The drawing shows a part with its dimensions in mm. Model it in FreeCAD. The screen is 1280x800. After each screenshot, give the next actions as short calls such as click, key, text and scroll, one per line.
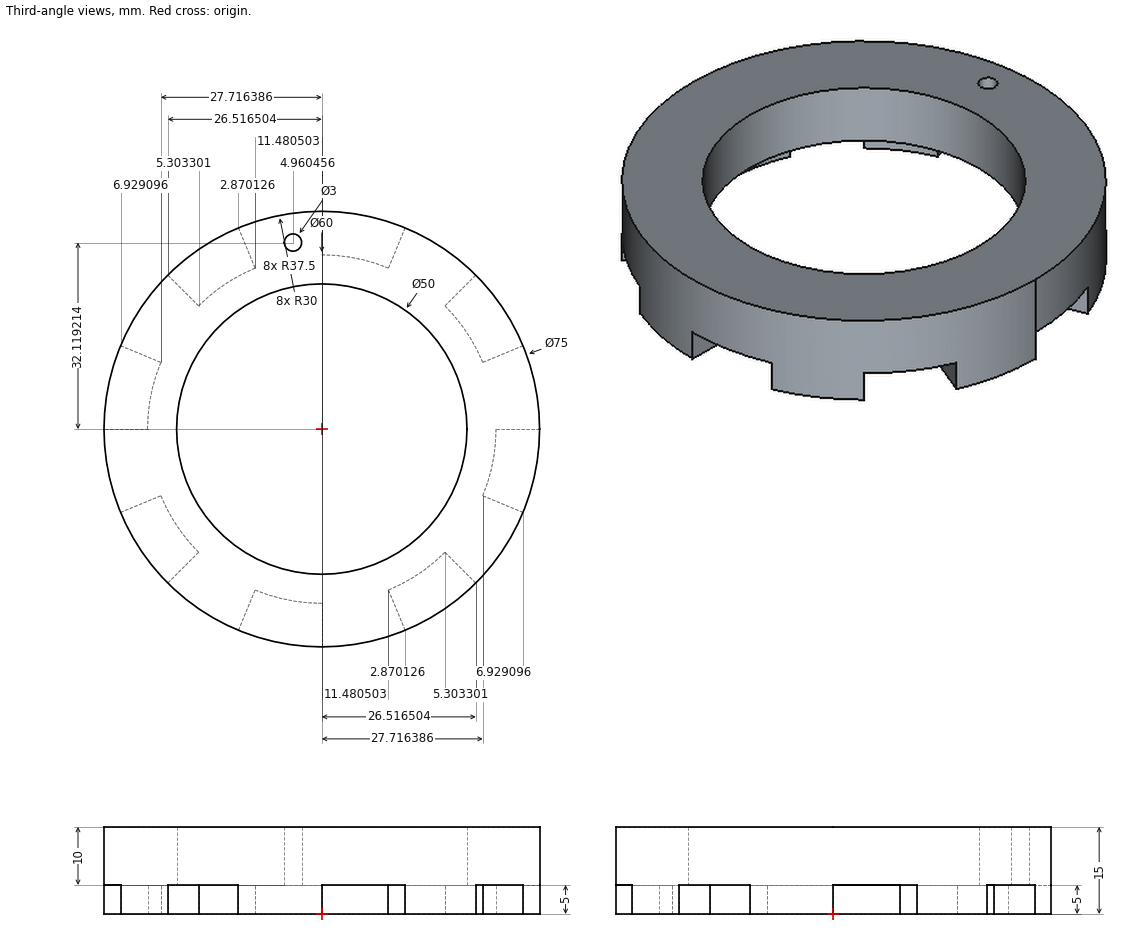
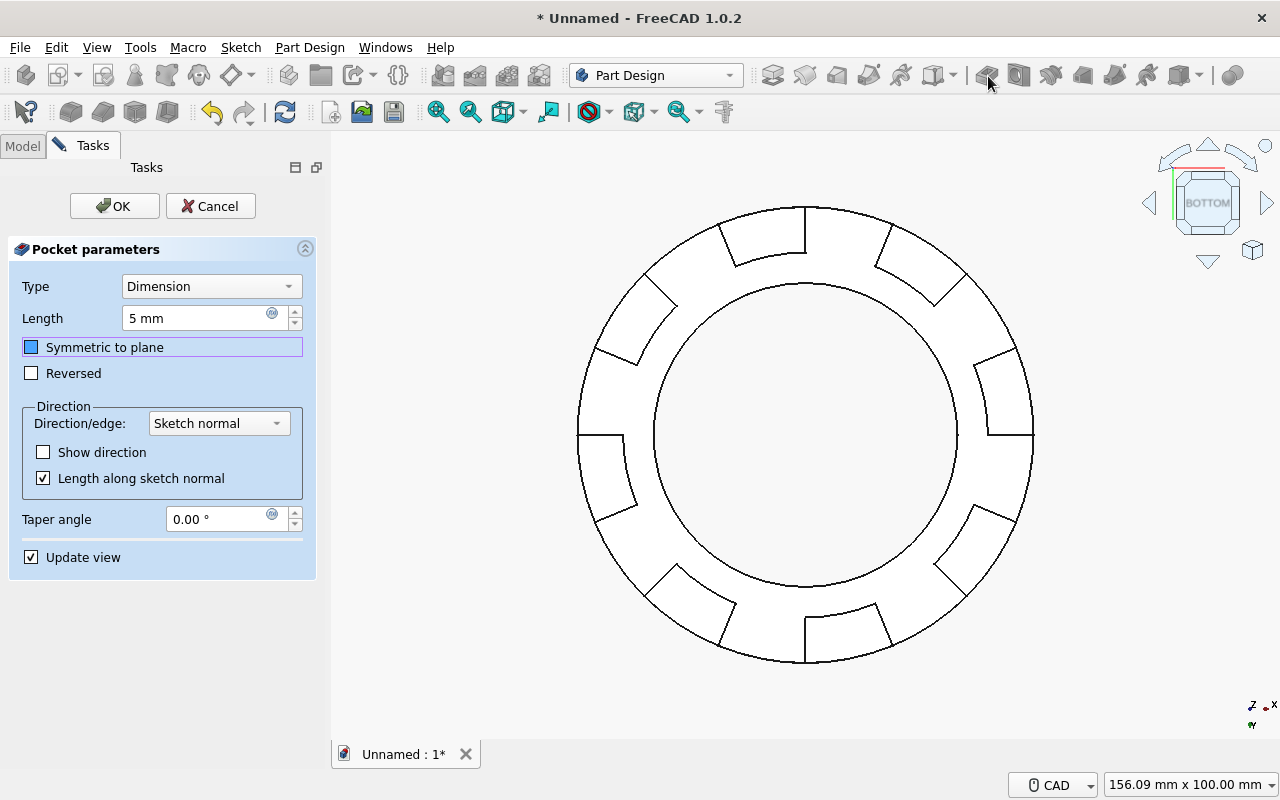
click(115, 206)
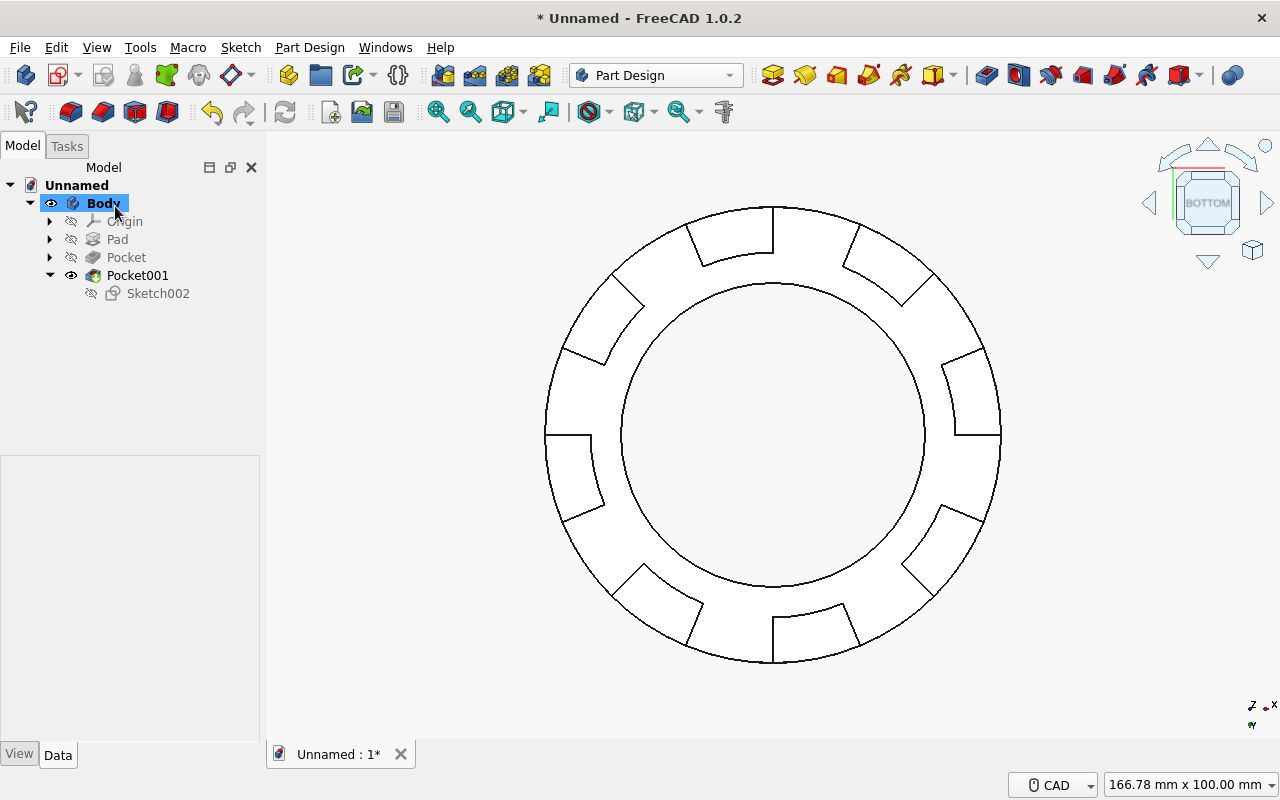
click(968, 499)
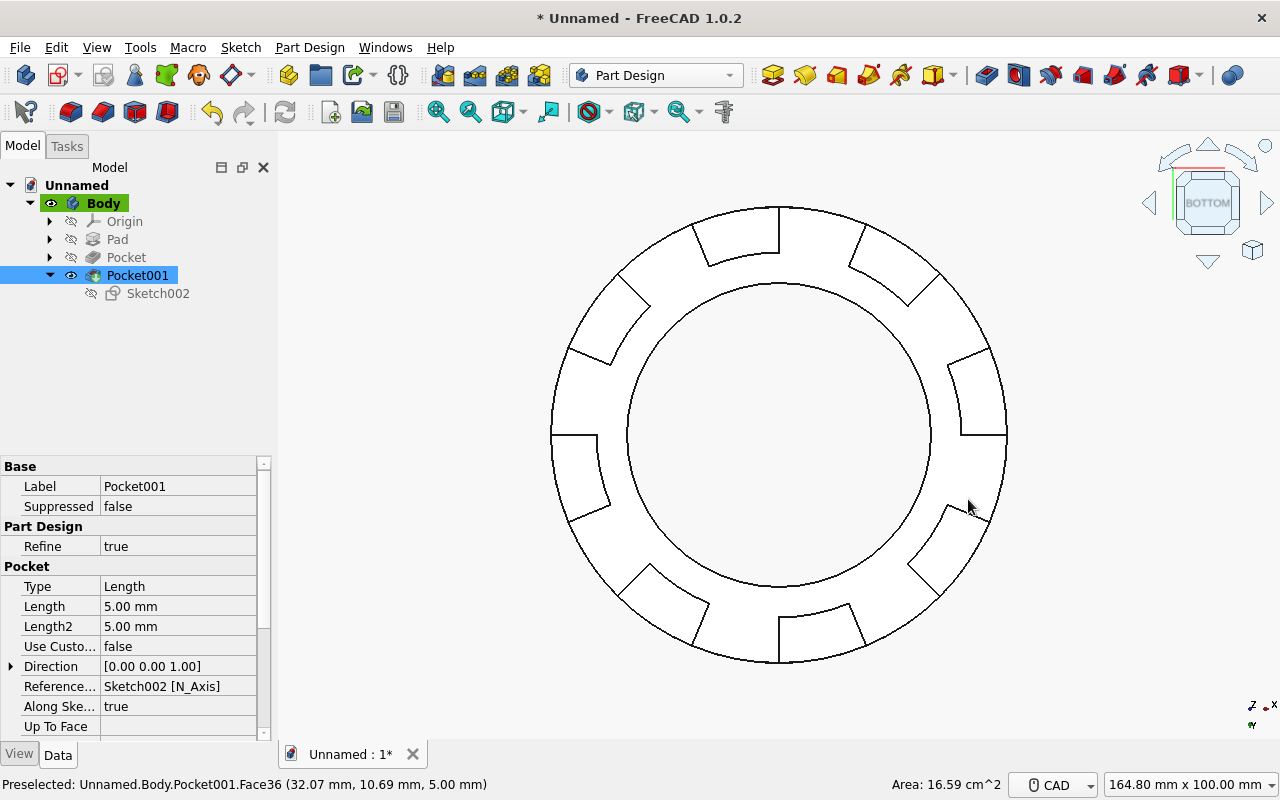
click(58, 76)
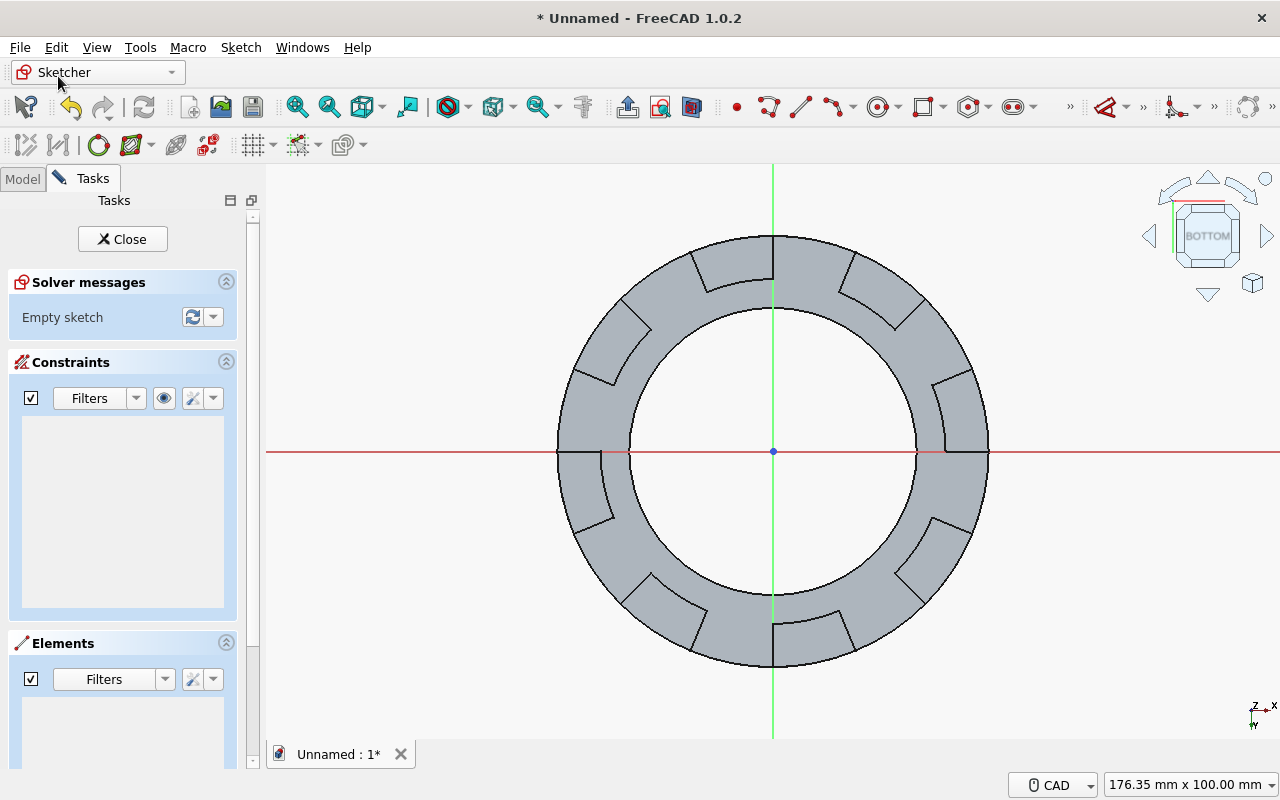
scroll(747, 646, up, 15)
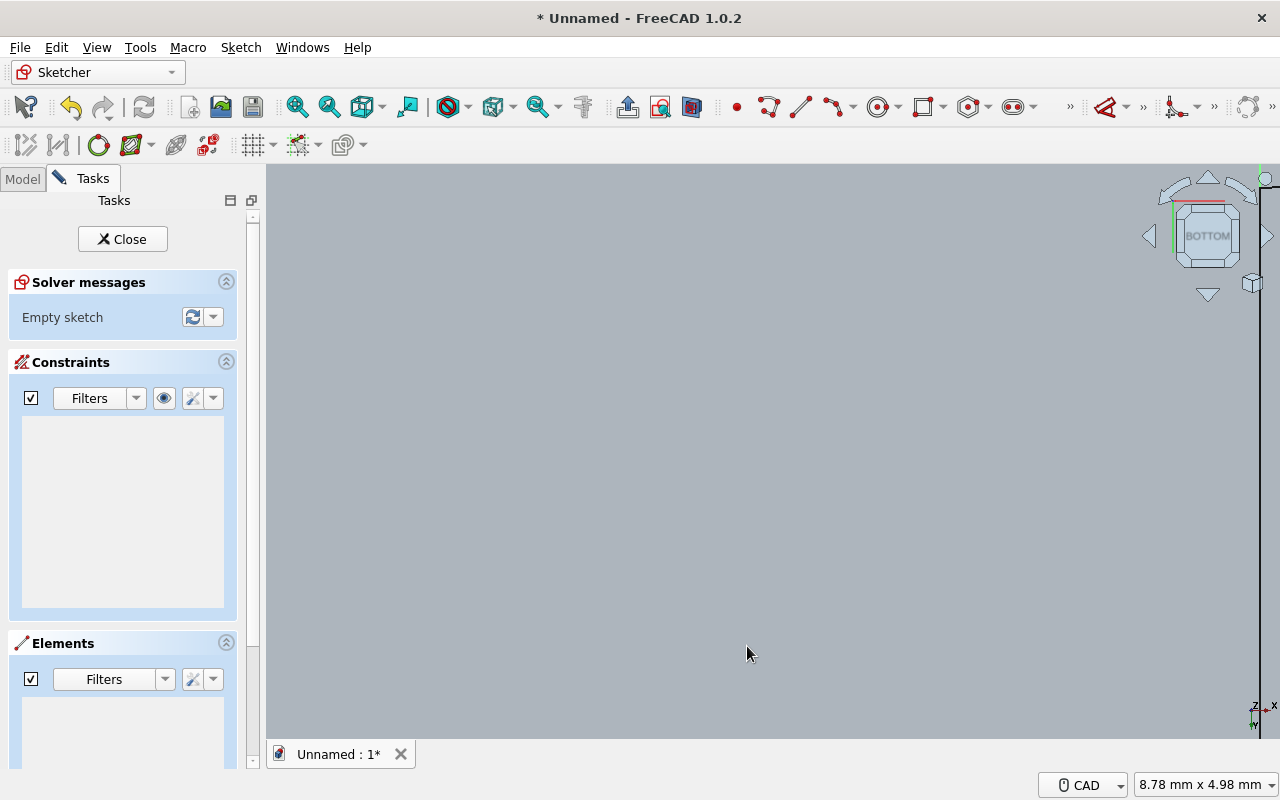
key(g)
key(c)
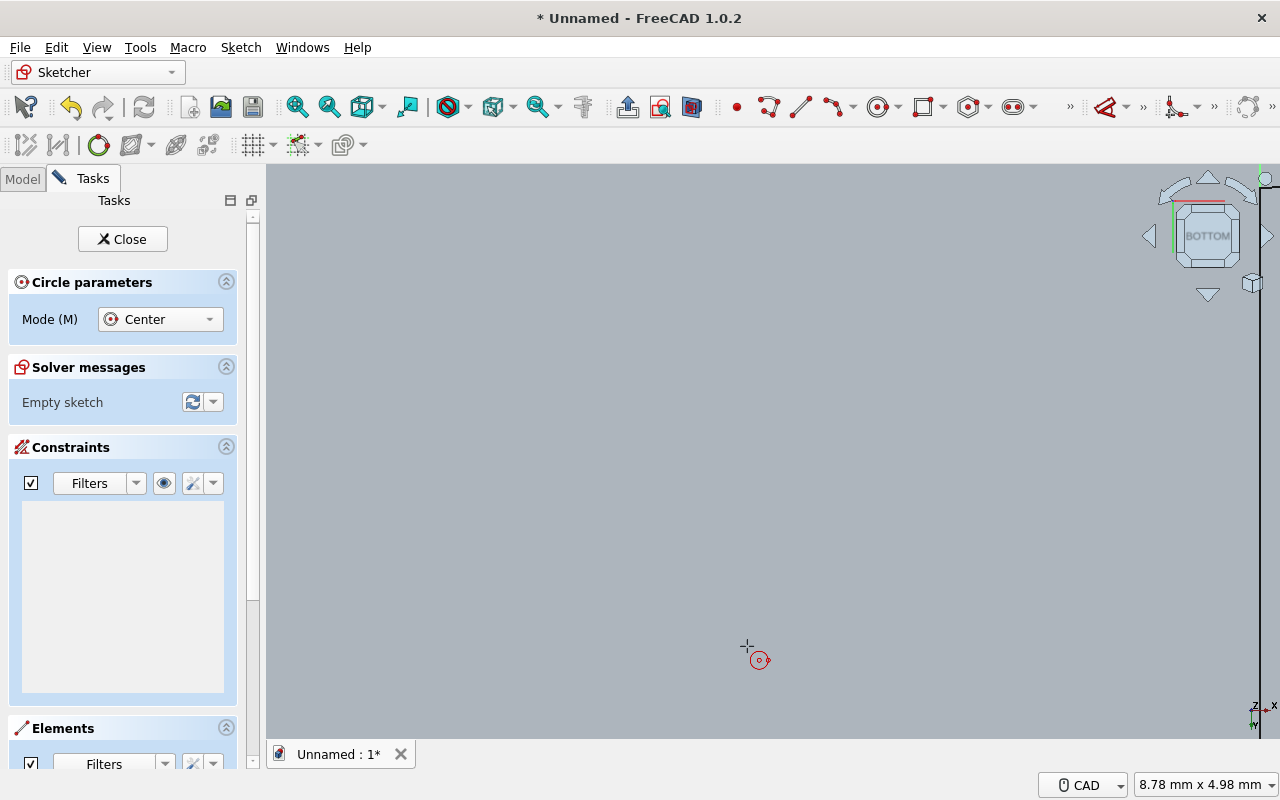
click(687, 433)
move(810, 310)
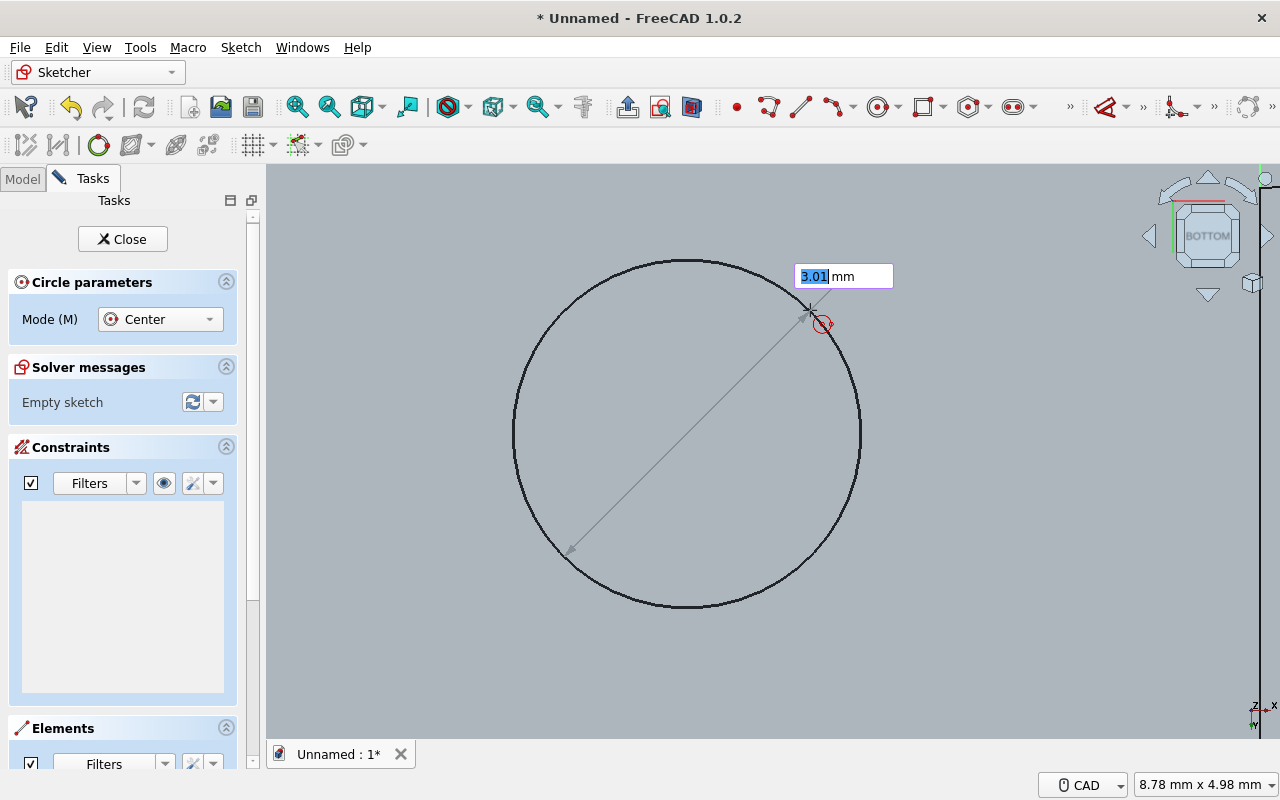
text(3)
key(Return)
key(Escape)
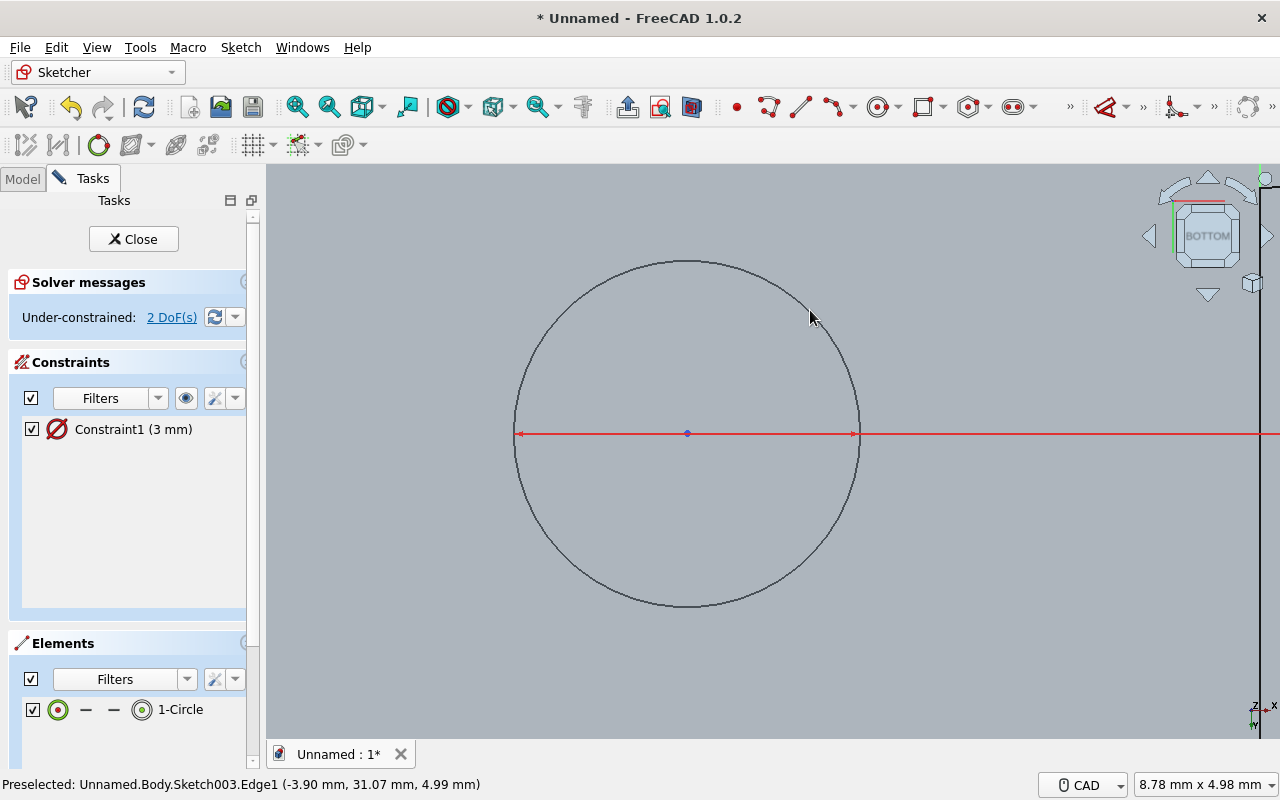
key(d)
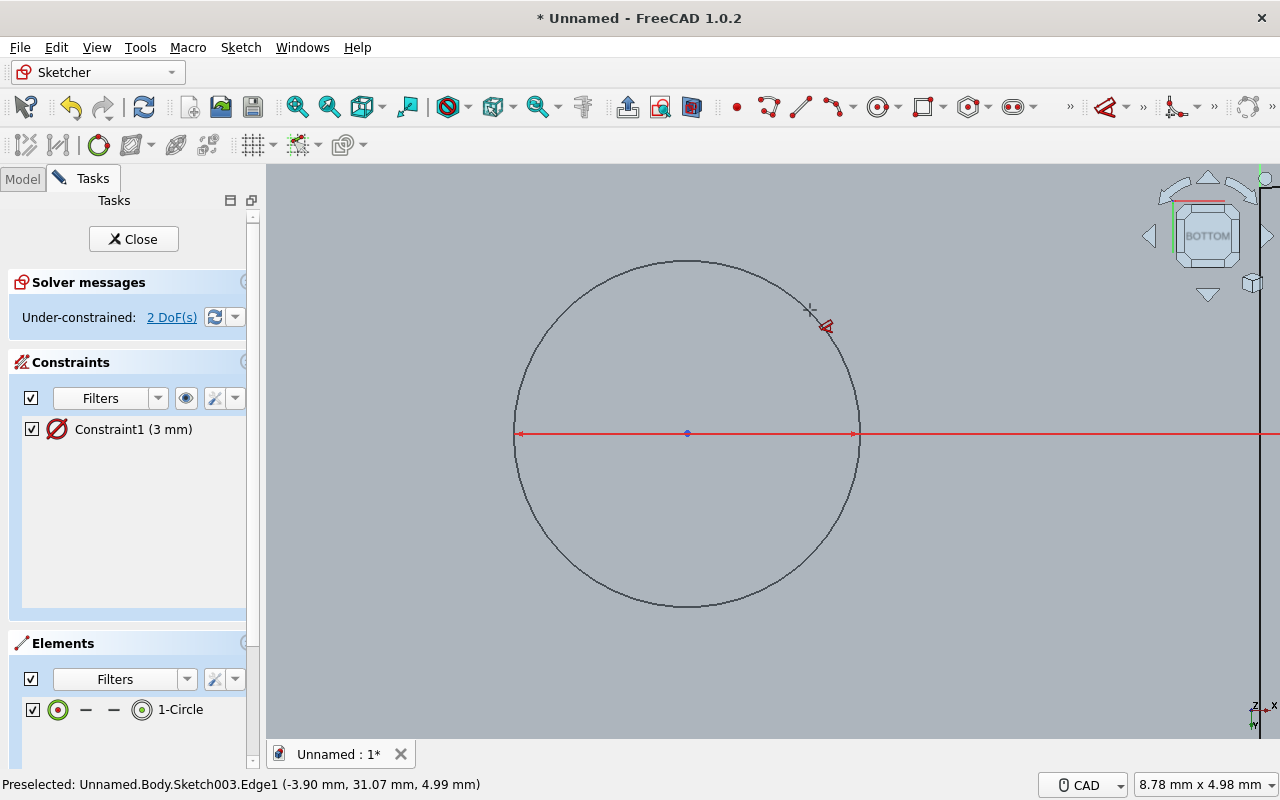
click(687, 434)
click(901, 468)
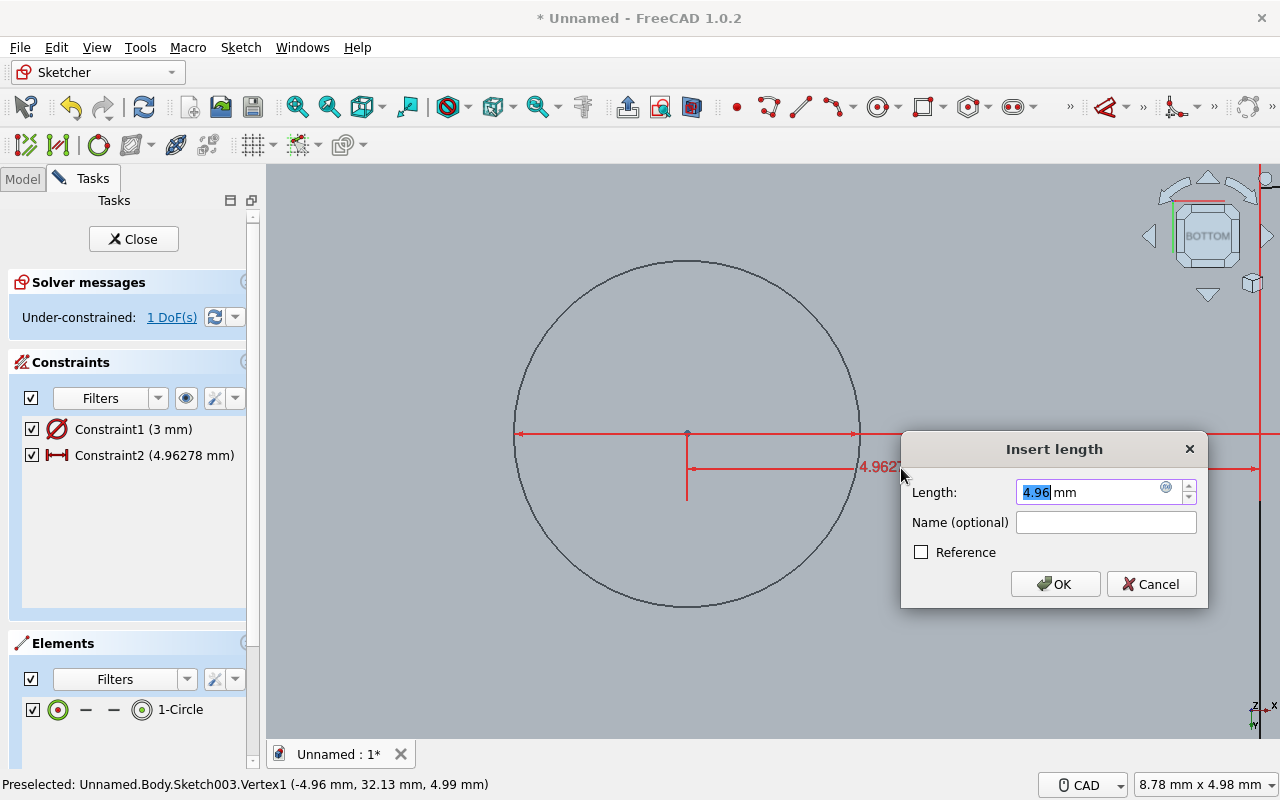
text(4.960456)
key(Return)